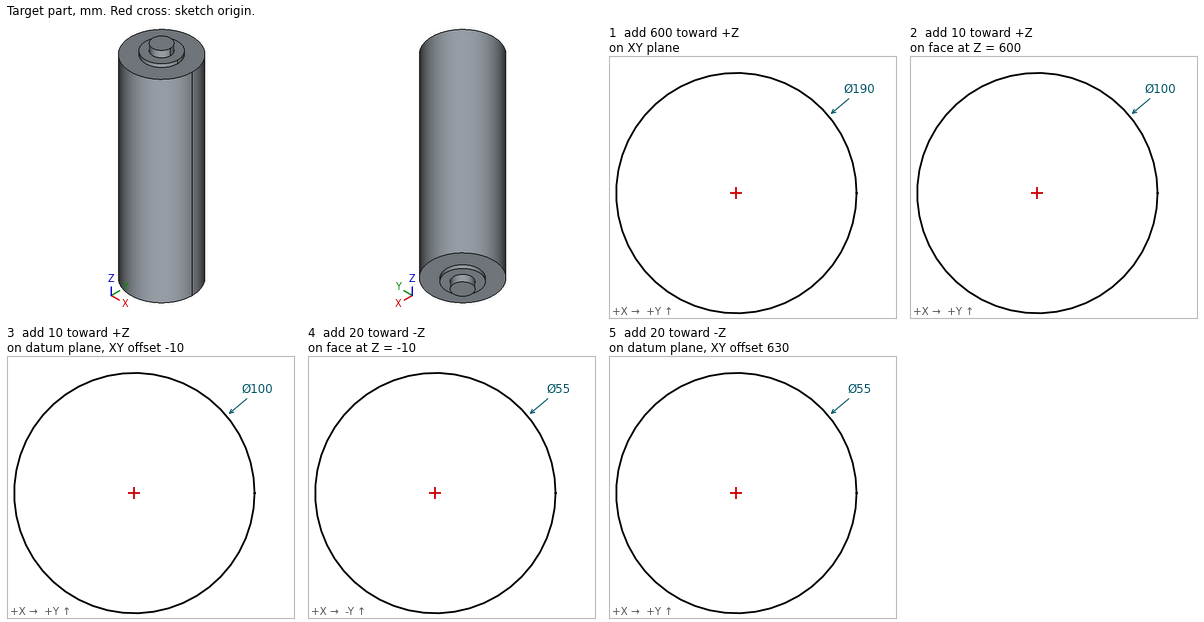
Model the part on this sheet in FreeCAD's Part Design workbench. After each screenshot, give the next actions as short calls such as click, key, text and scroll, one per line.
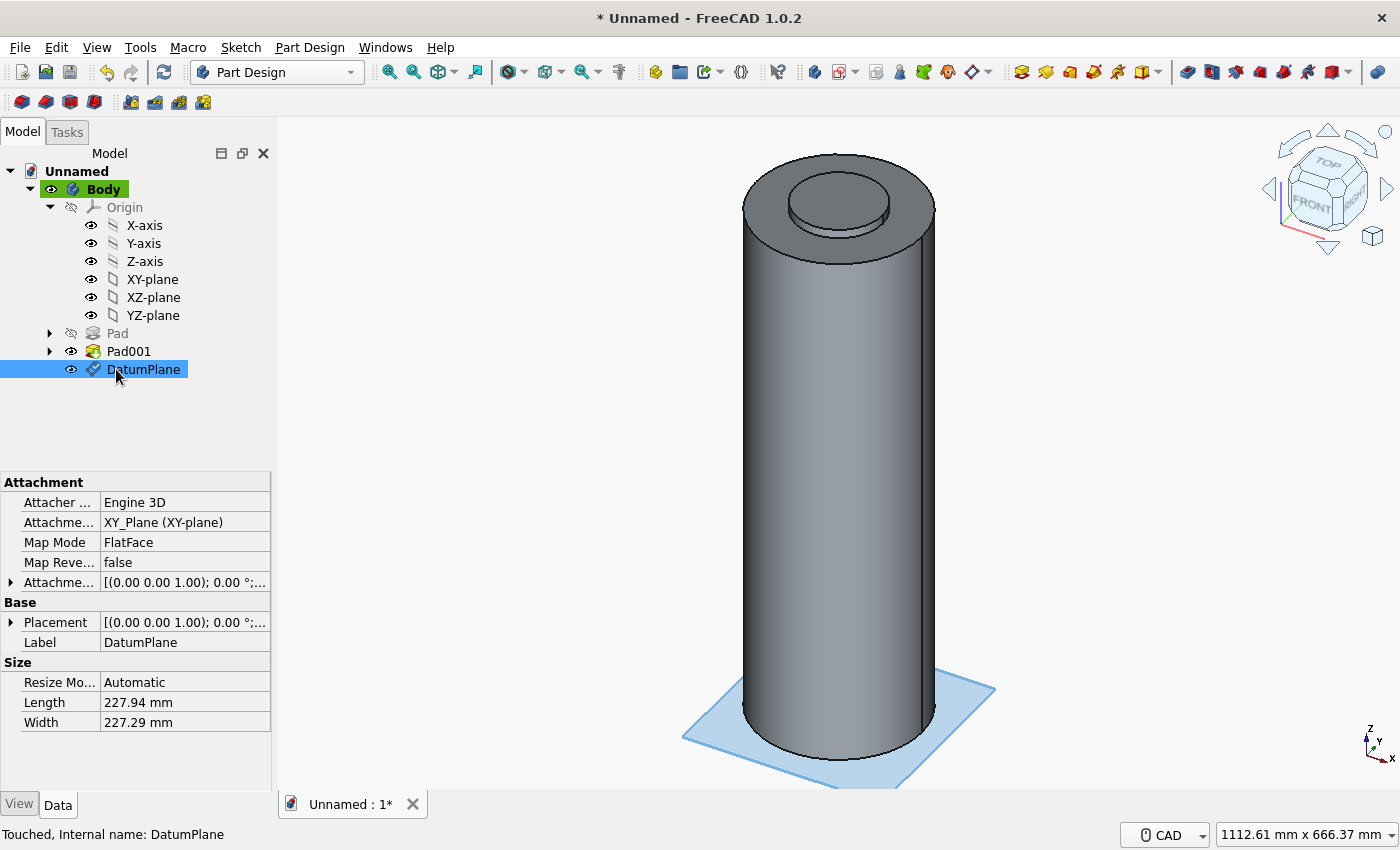
click(840, 72)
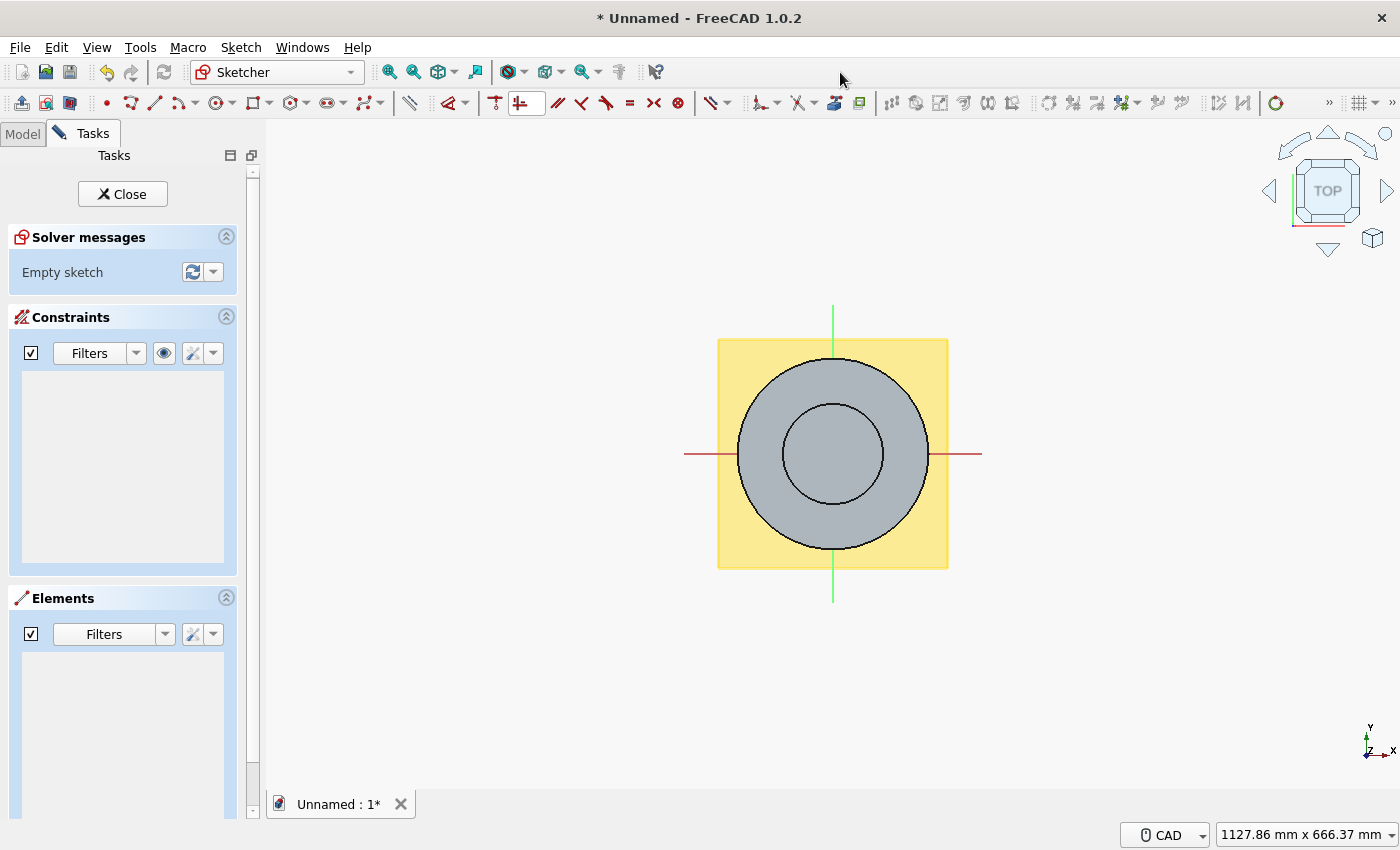
click(70, 104)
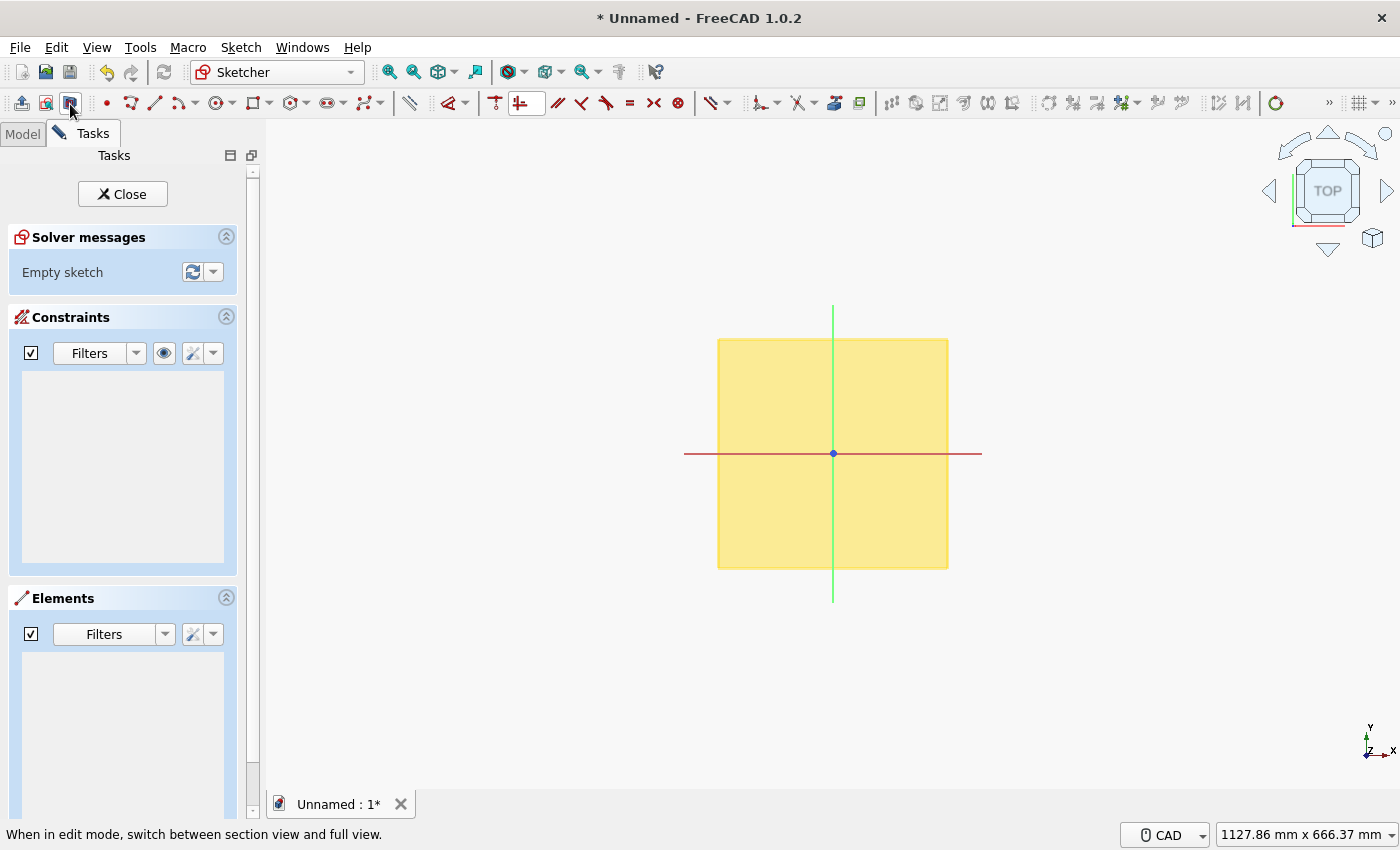
scroll(855, 454, up, 7)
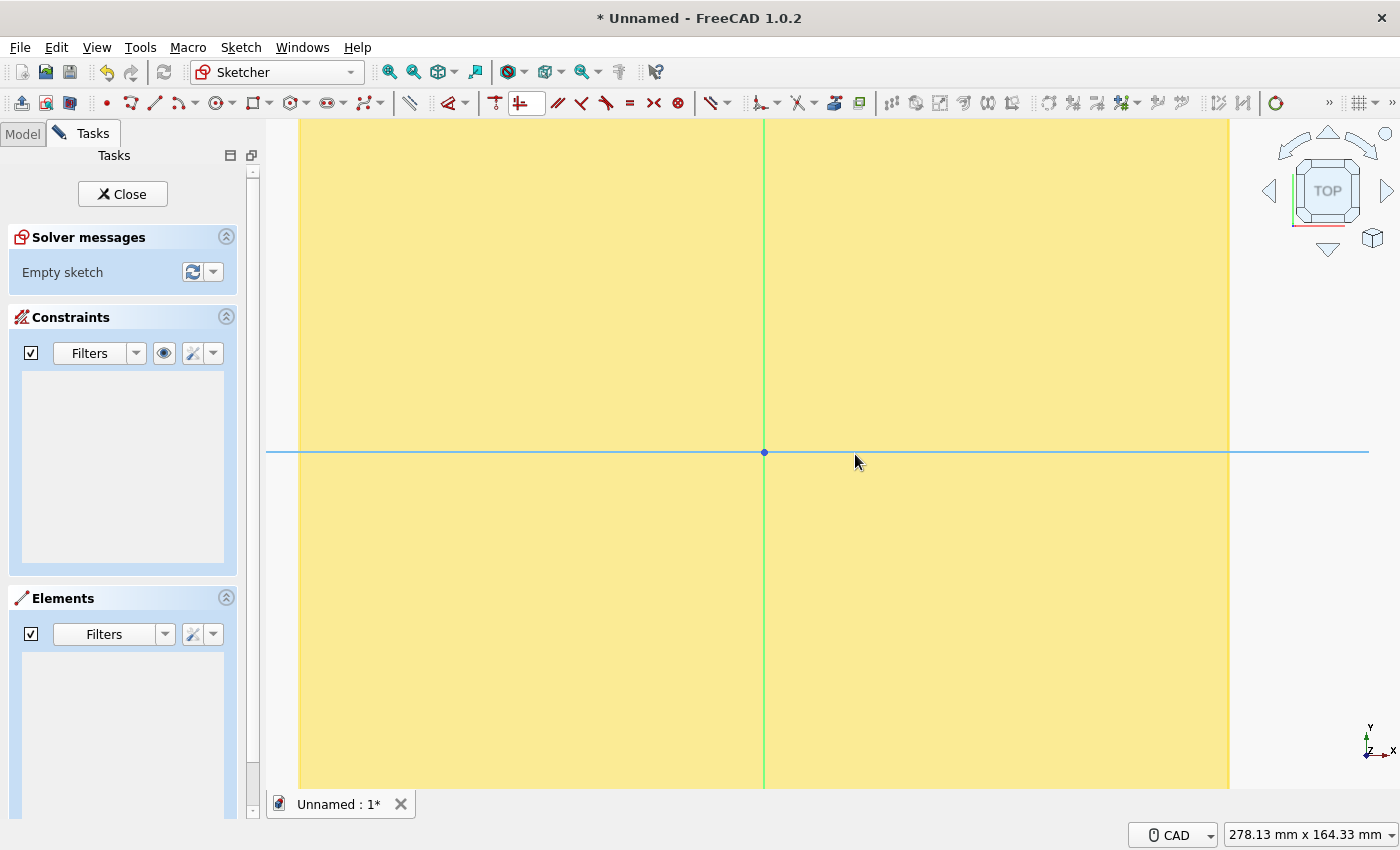
click(216, 104)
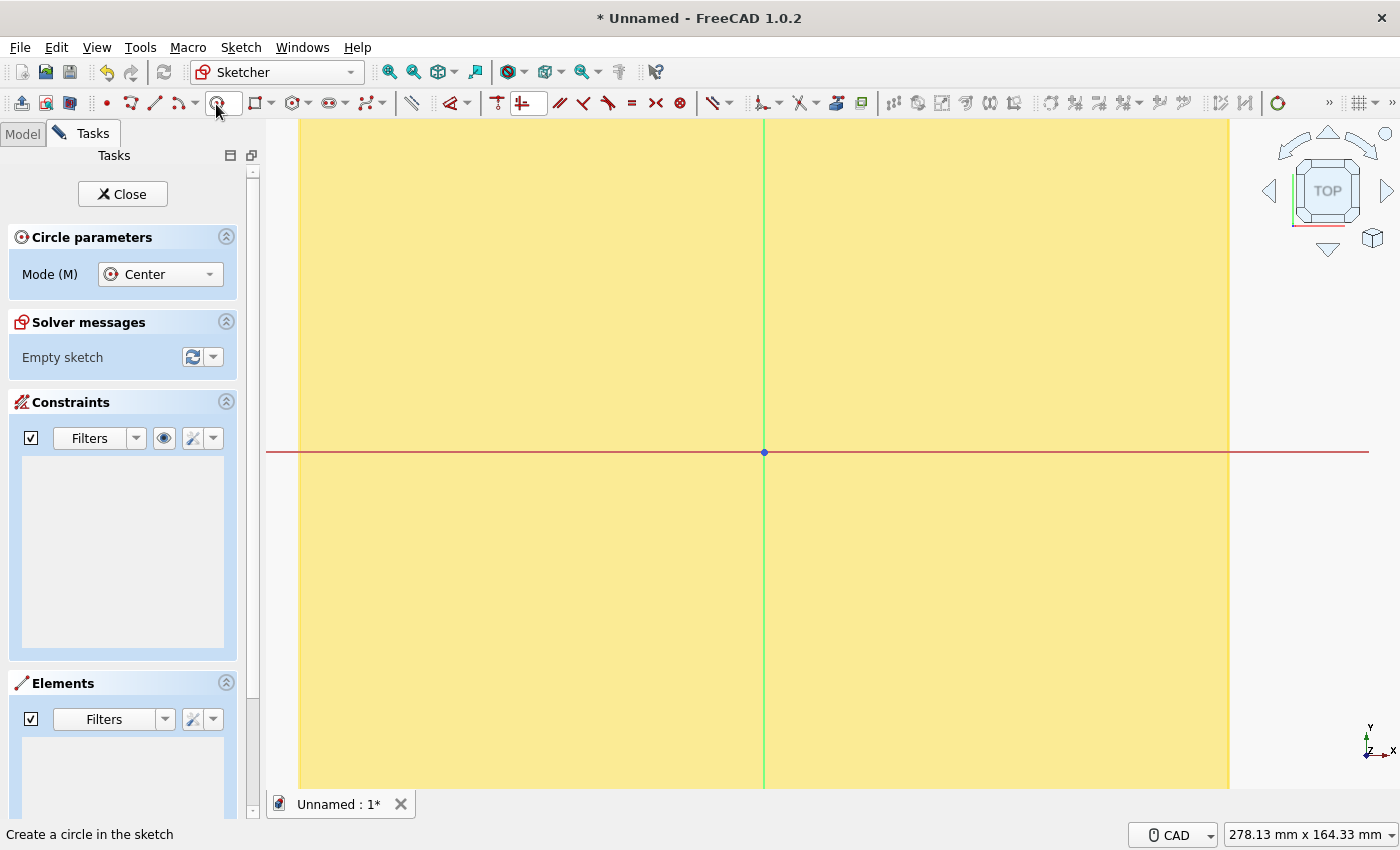
click(764, 452)
click(908, 308)
key(Escape)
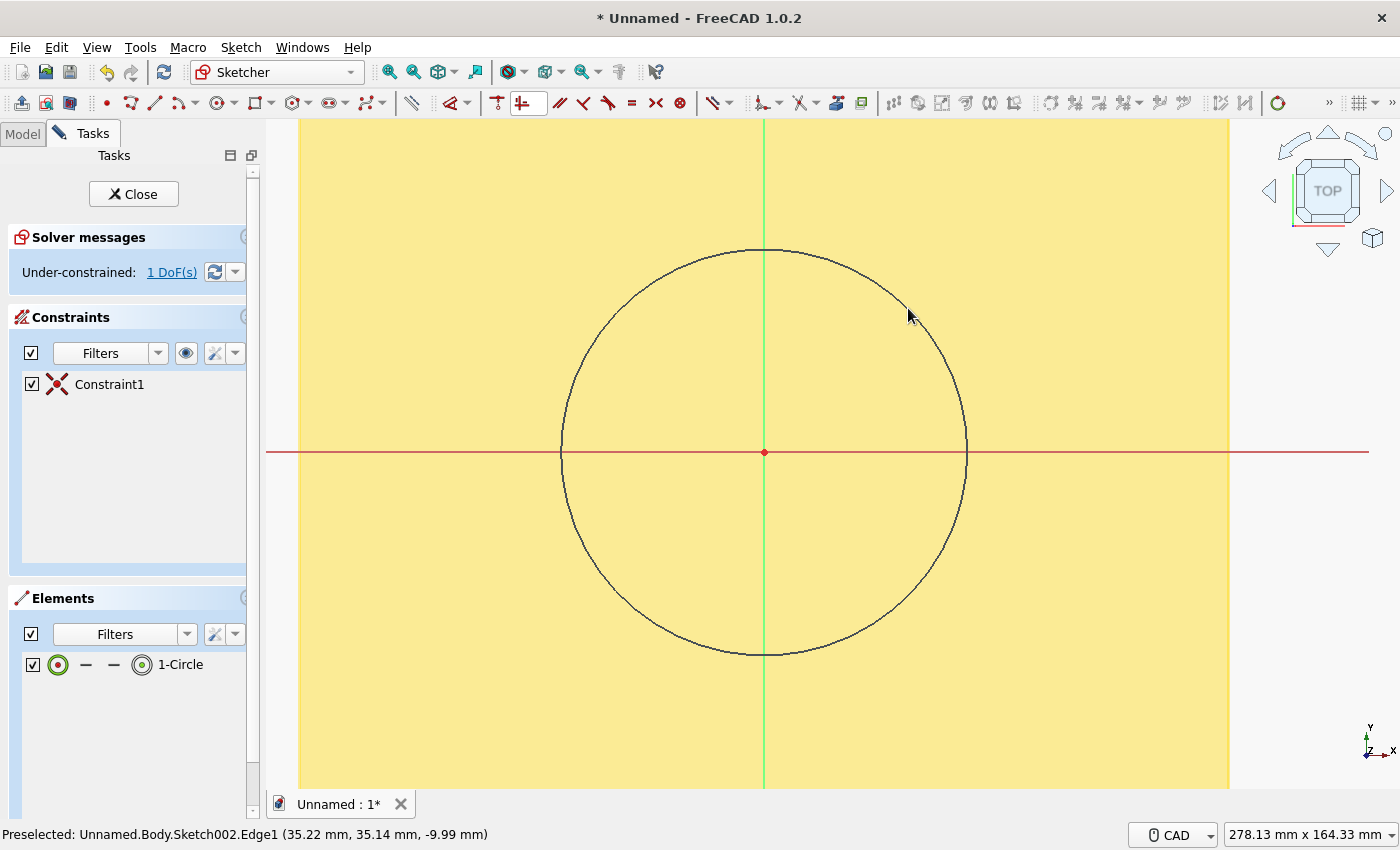
click(450, 104)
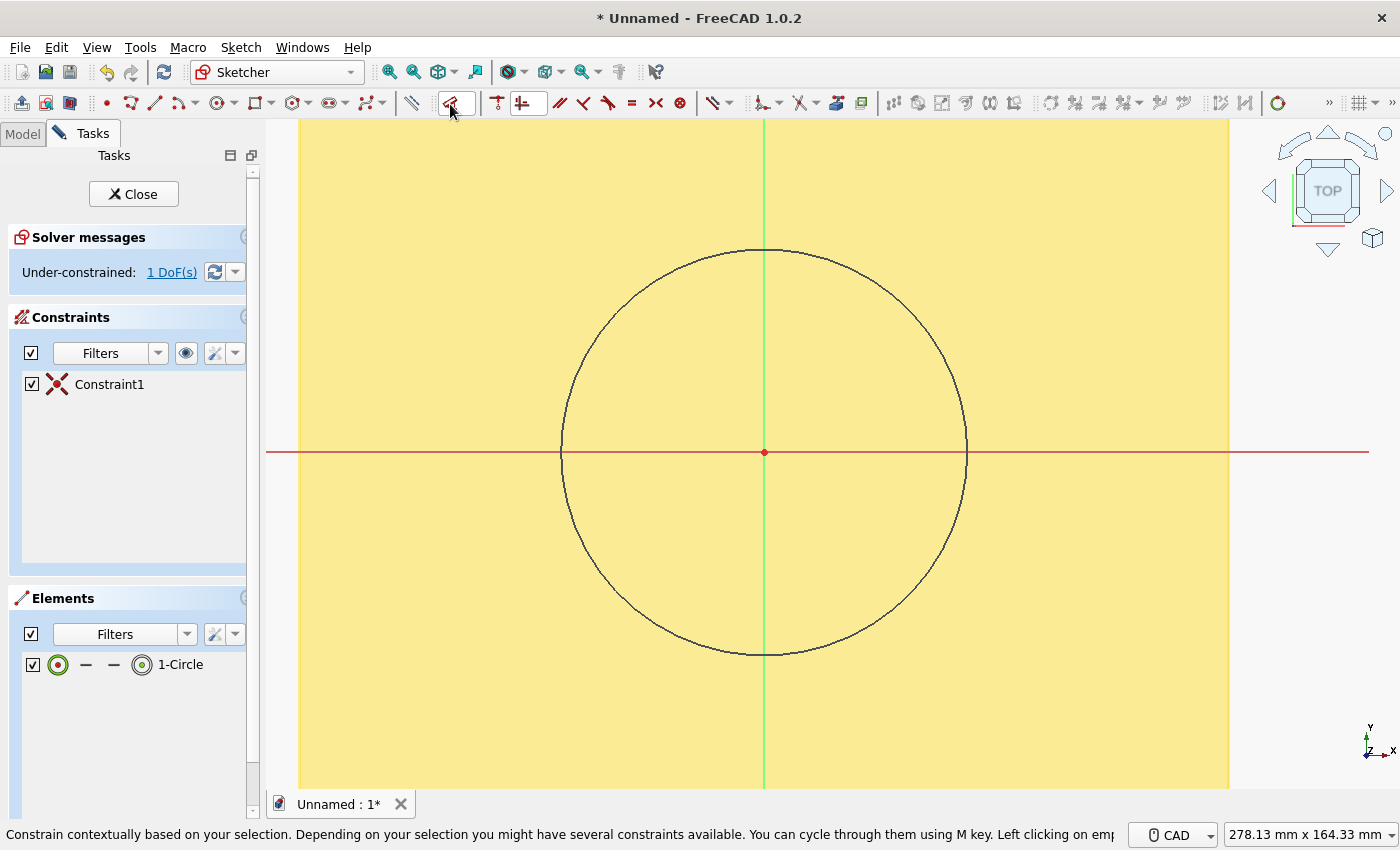
click(907, 308)
click(929, 285)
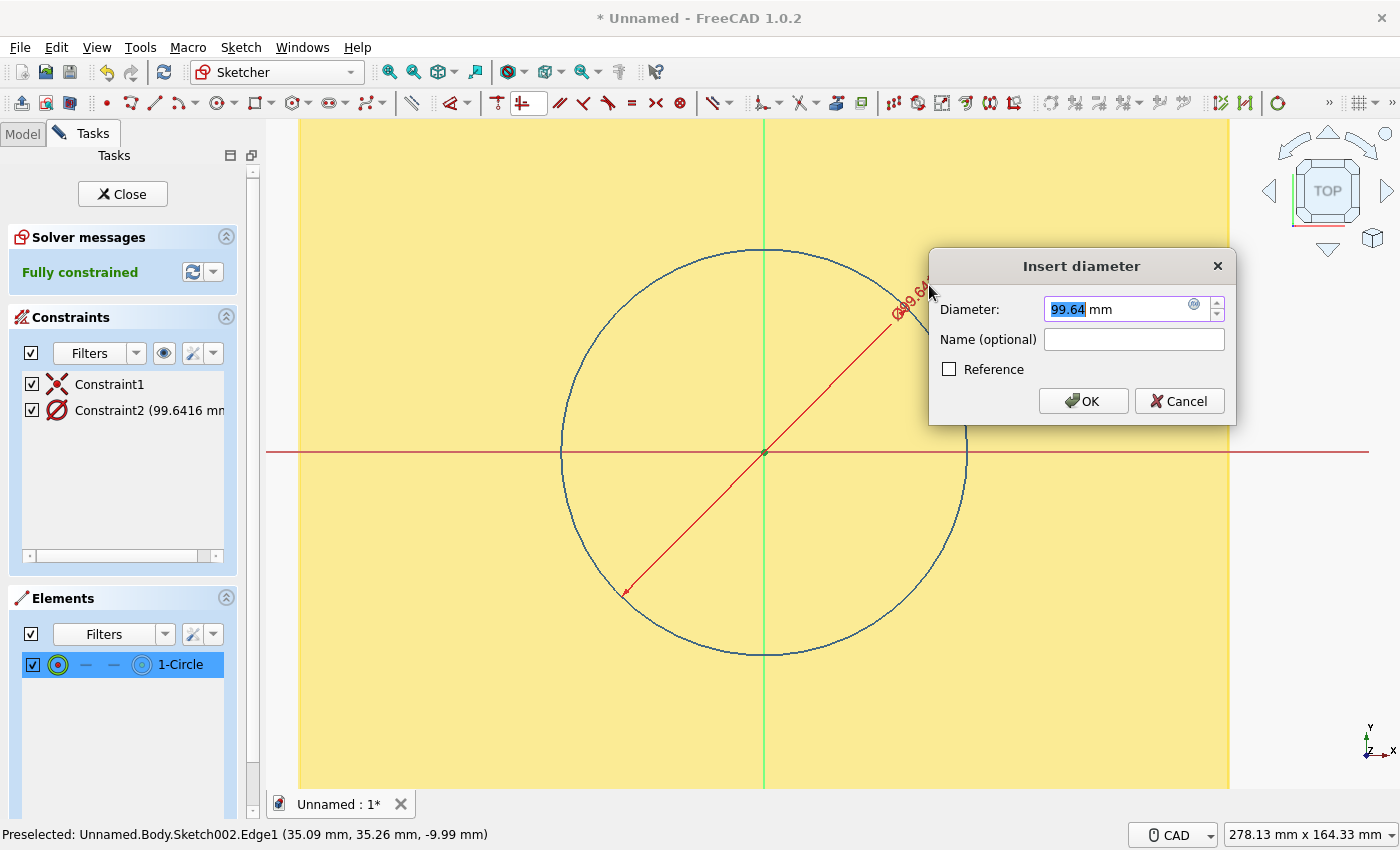
text(100)
key(Return)
key(Escape)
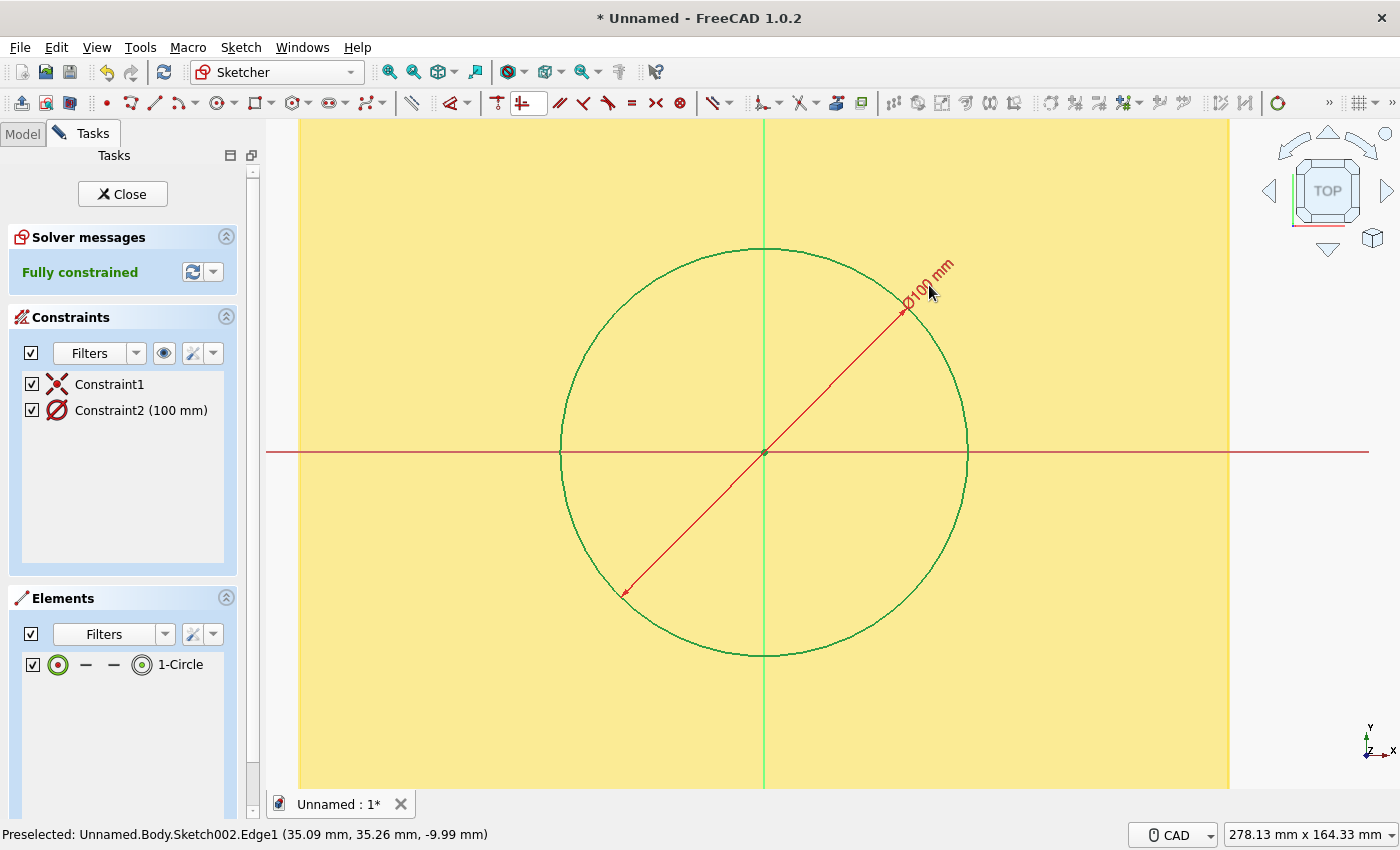
click(123, 194)